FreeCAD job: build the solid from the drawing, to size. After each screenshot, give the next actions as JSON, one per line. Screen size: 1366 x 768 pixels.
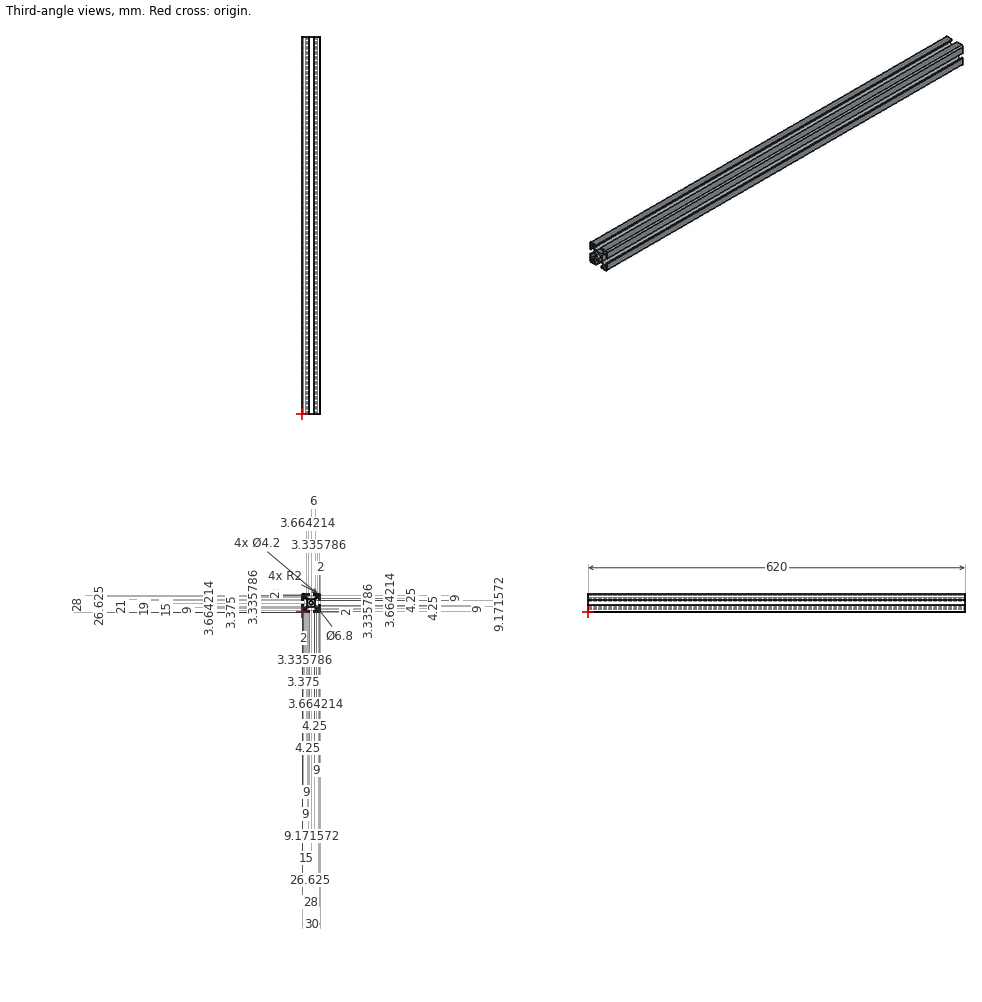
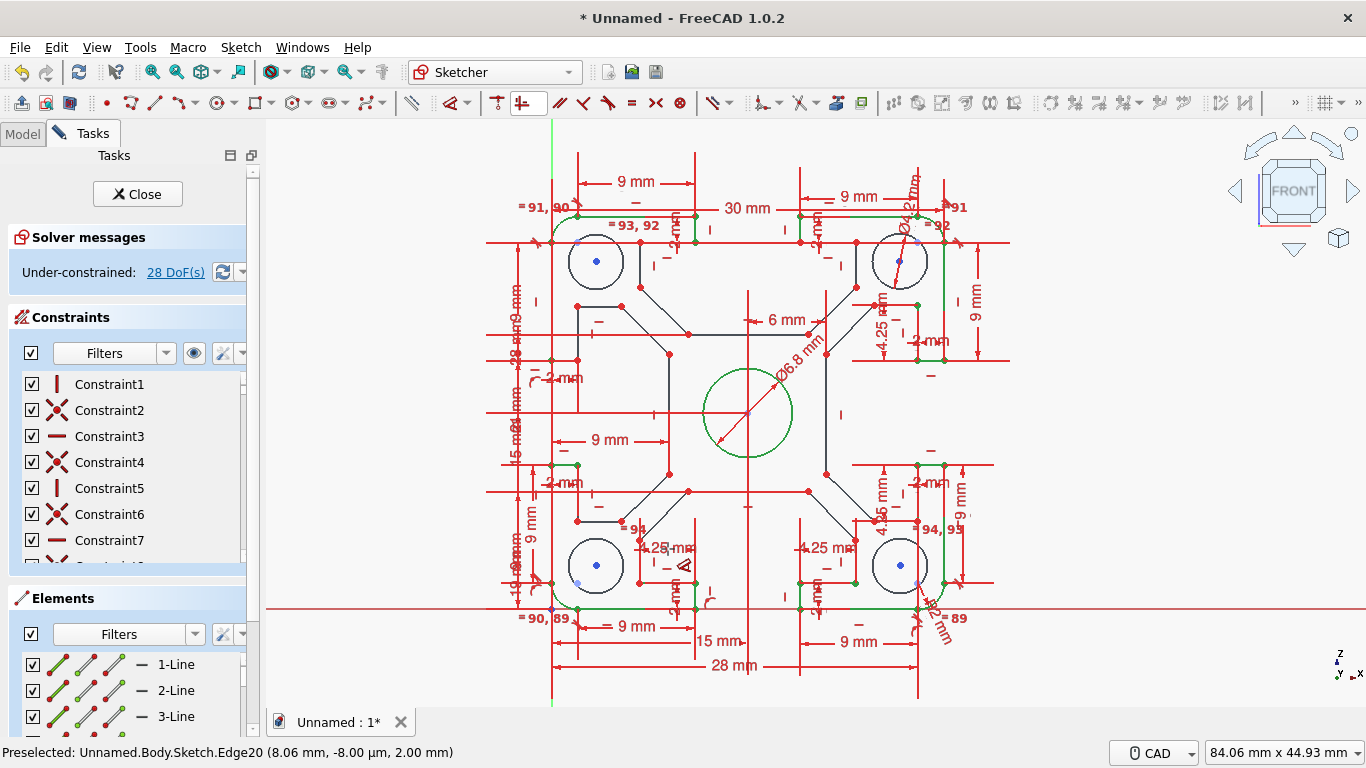
{"action": "left_click", "coordinate": [578, 482]}
{"action": "left_click", "coordinate": [612, 506]}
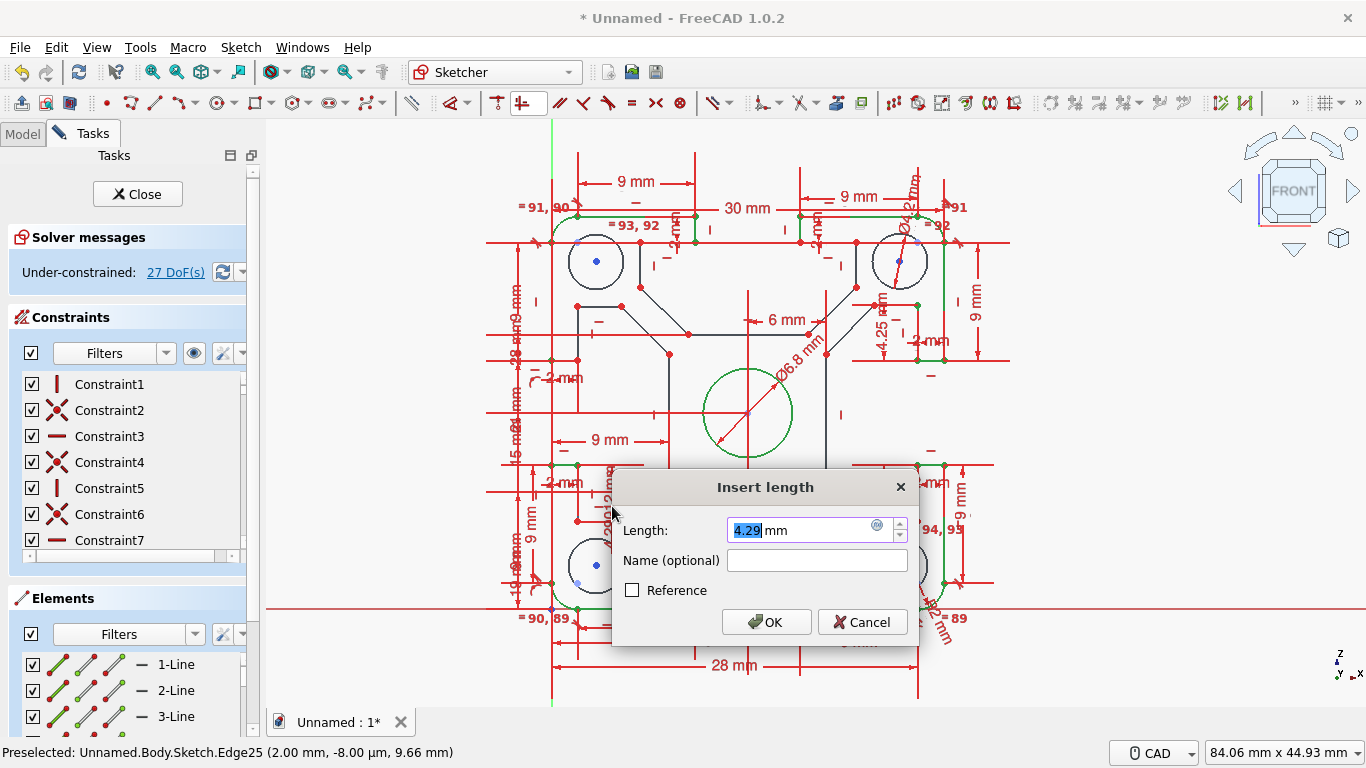
{"action": "type", "text": "4.25"}
{"action": "key", "text": "Return"}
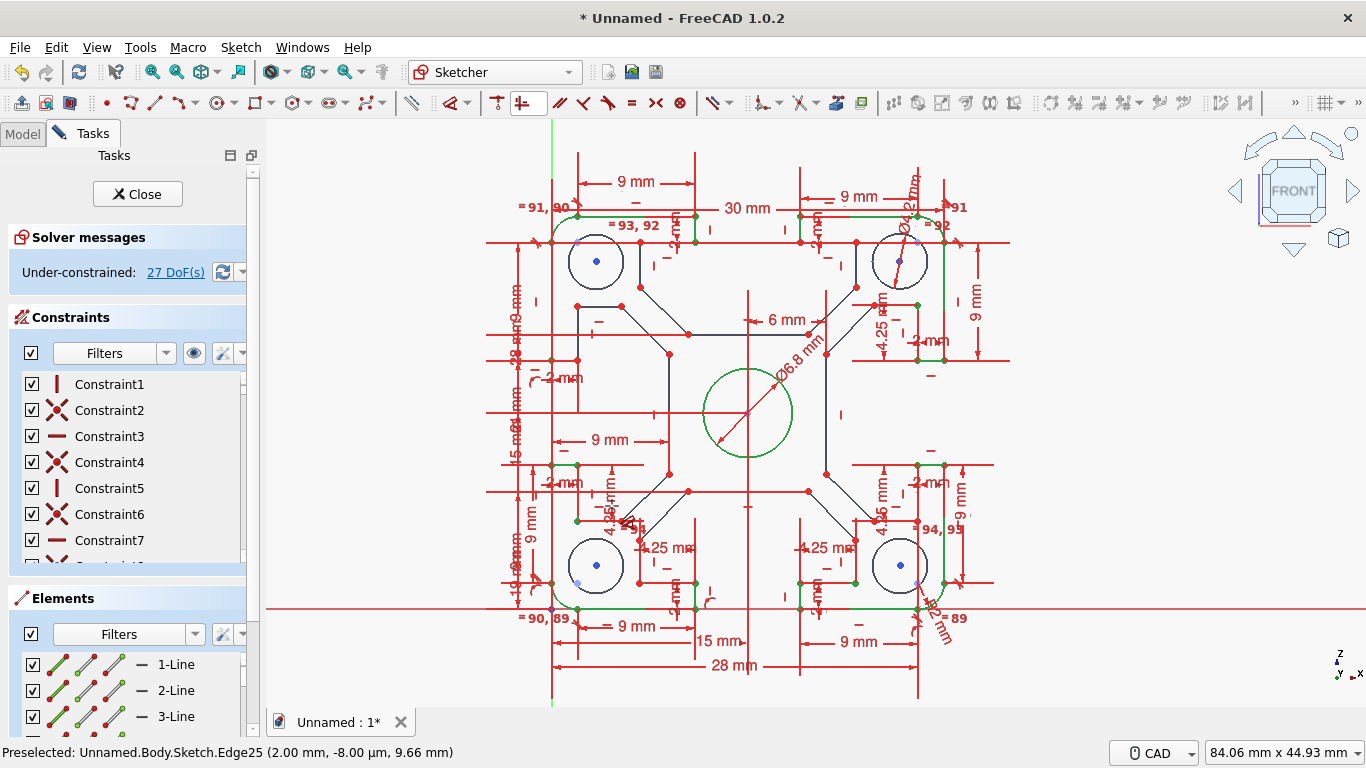
{"action": "left_click", "coordinate": [578, 323]}
{"action": "left_click", "coordinate": [612, 334]}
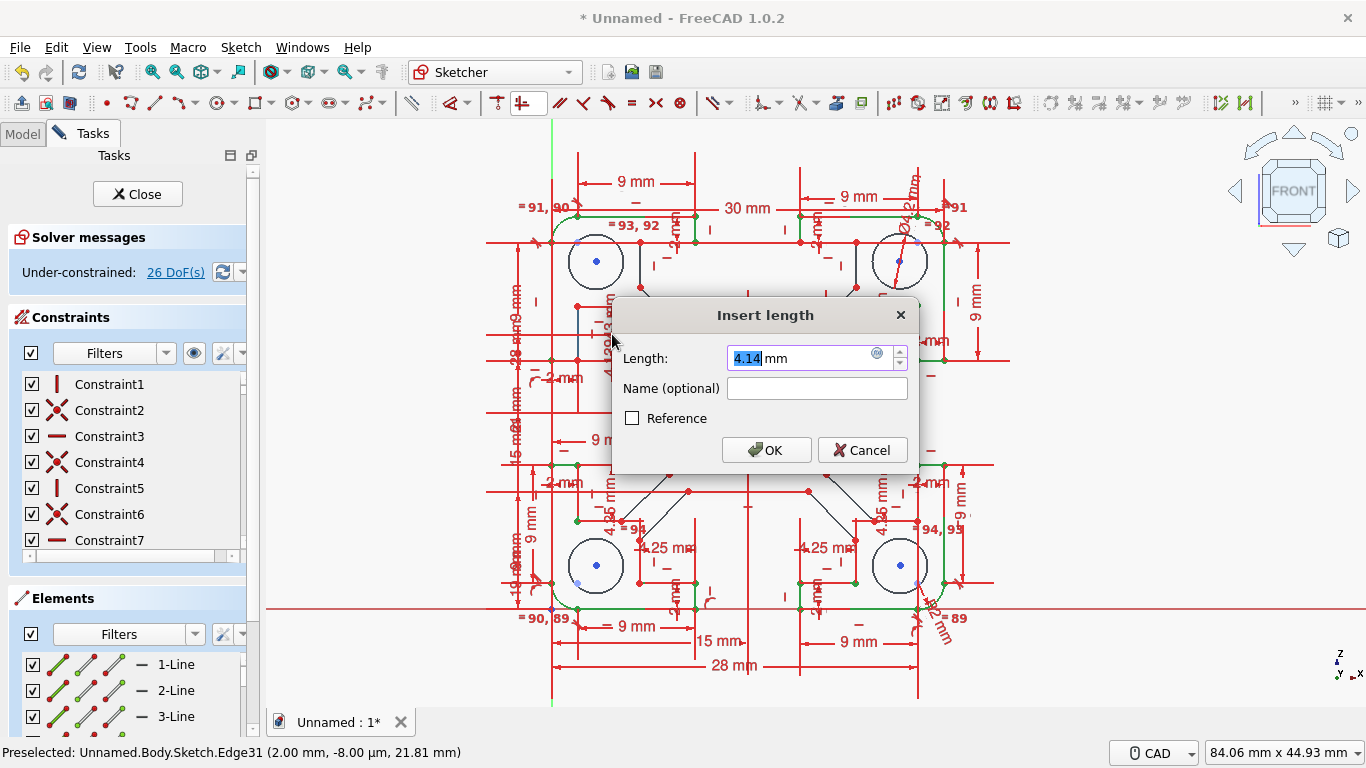
{"action": "type", "text": "4.25"}
{"action": "key", "text": "Return"}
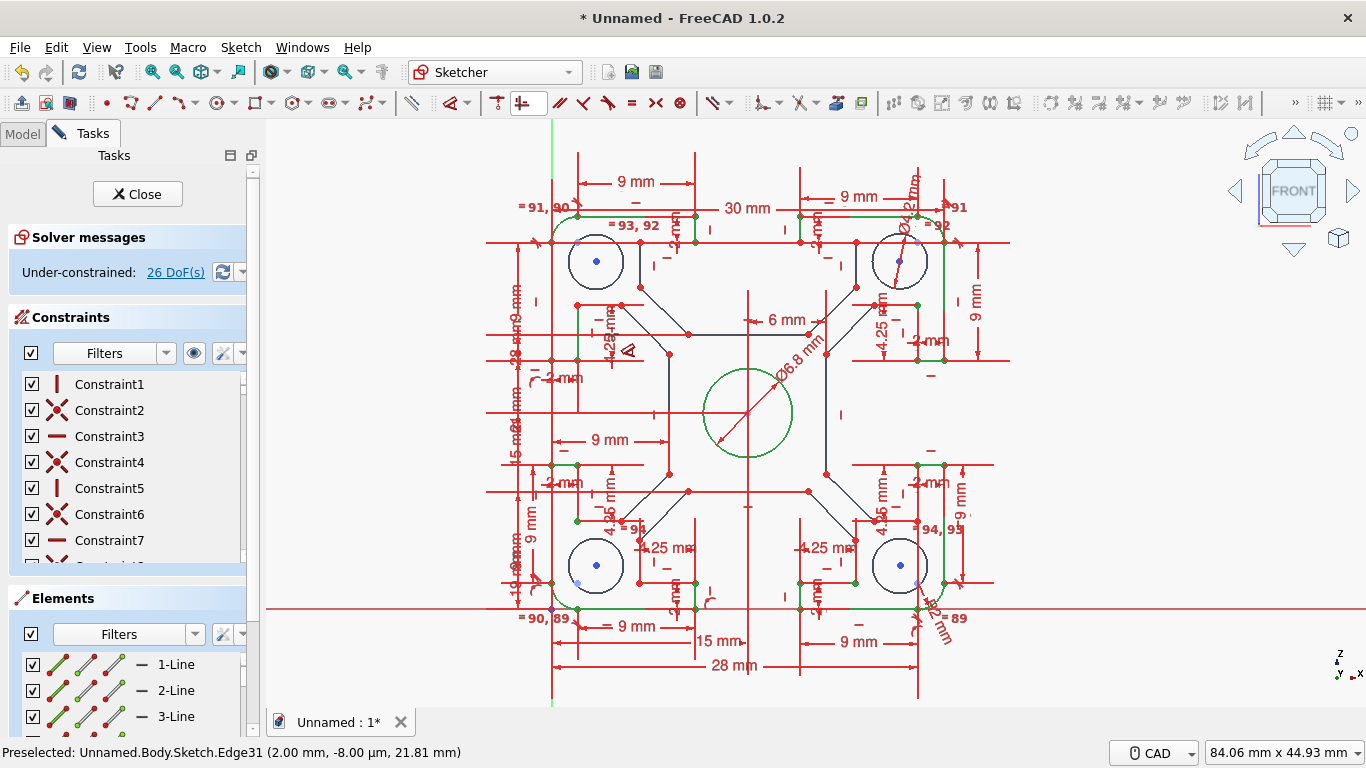
{"action": "left_click", "coordinate": [679, 243]}
{"action": "left_click", "coordinate": [668, 277]}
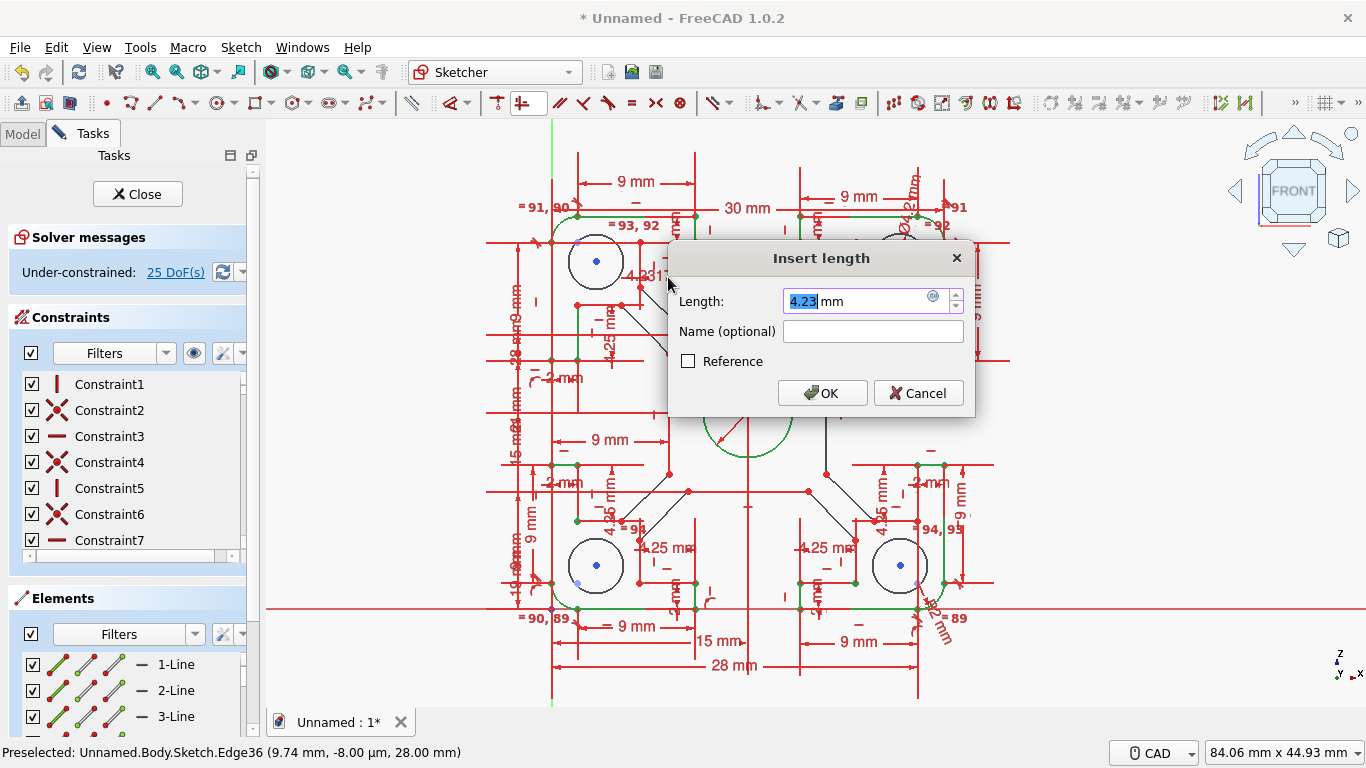
{"action": "type", "text": "4.25"}
{"action": "key", "text": "Return"}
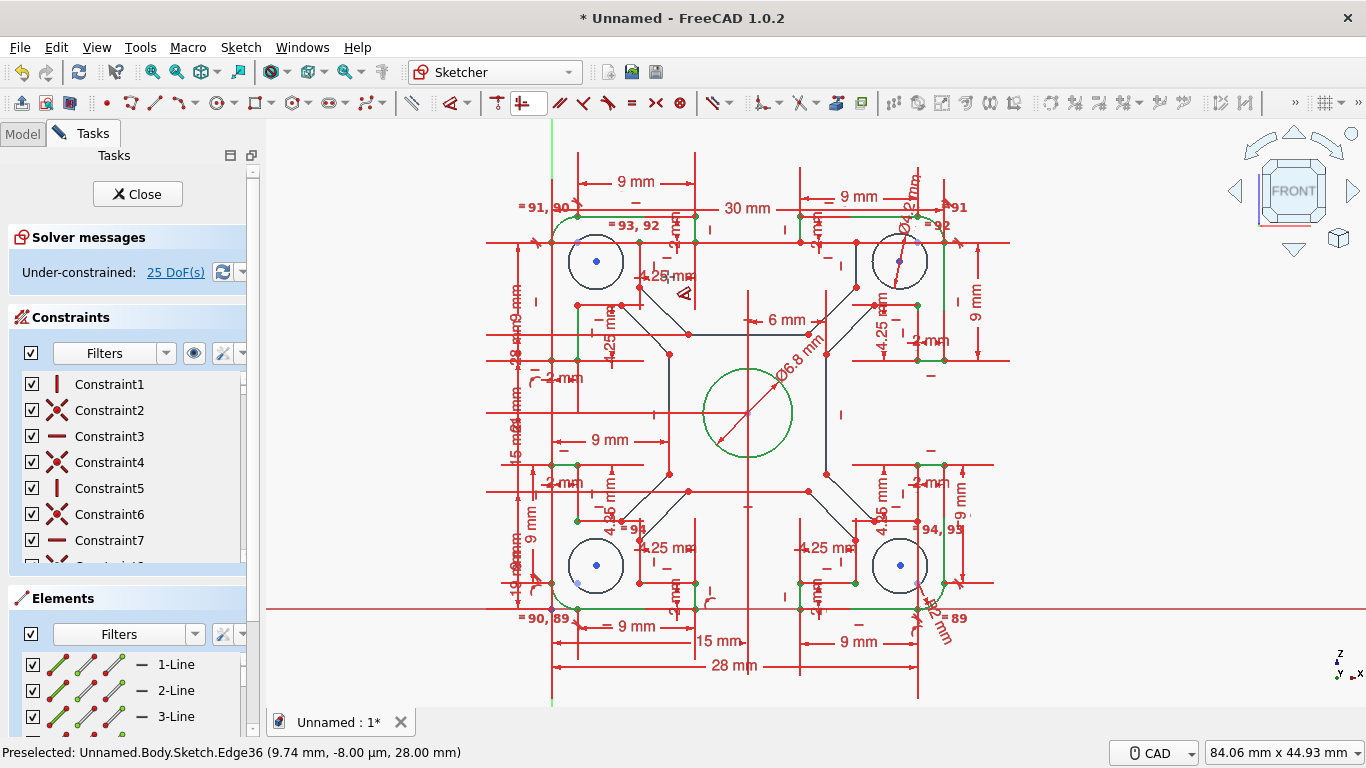
{"action": "left_click", "coordinate": [839, 243]}
{"action": "left_click", "coordinate": [828, 277]}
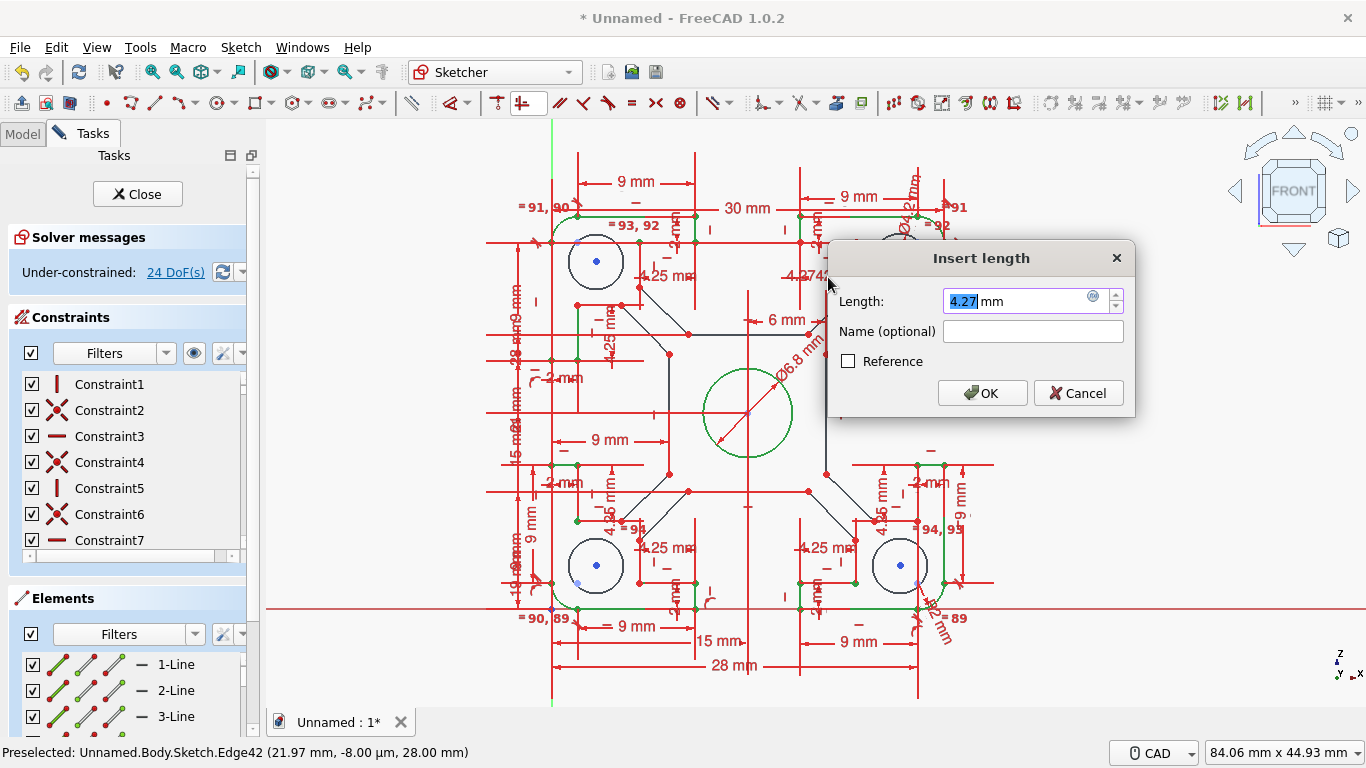
{"action": "type", "text": "4.25"}
{"action": "key", "text": "Return"}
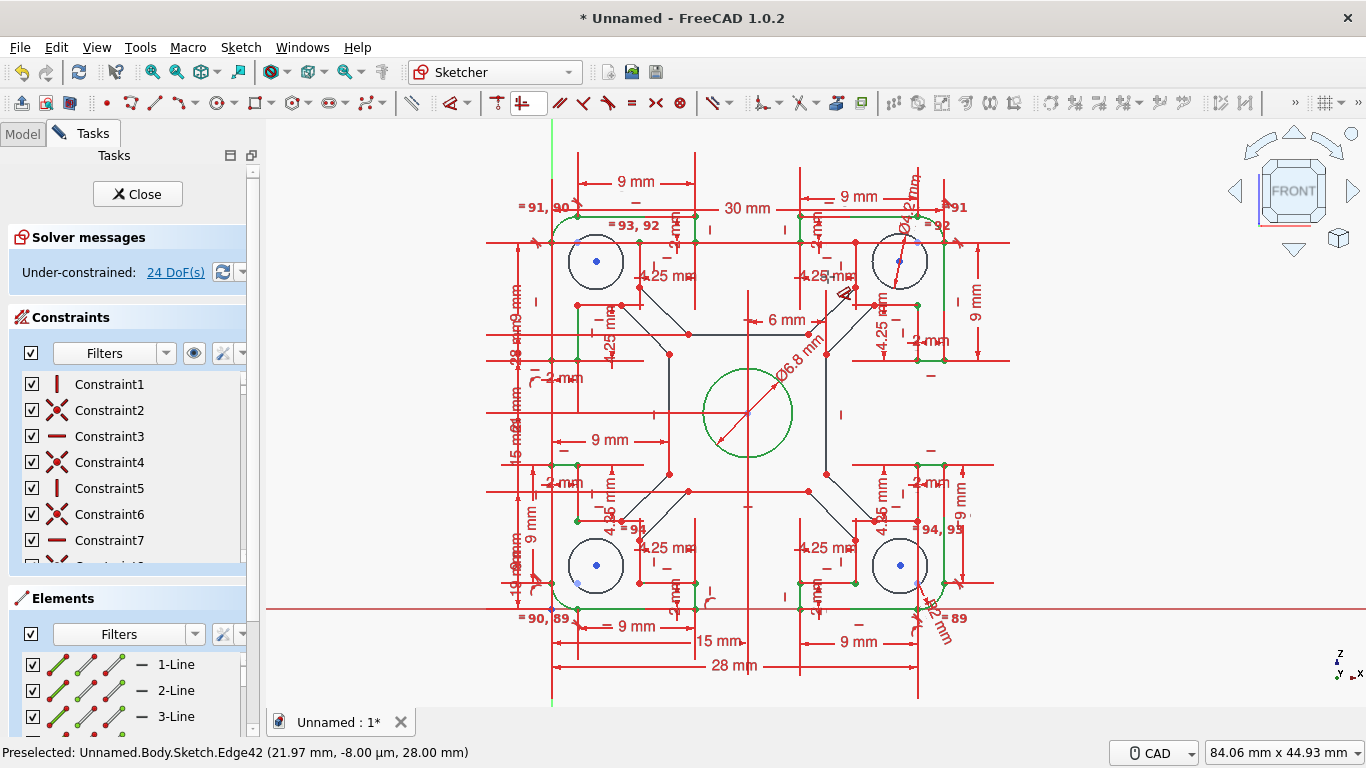
{"action": "left_click", "coordinate": [596, 262]}
{"action": "left_click", "coordinate": [574, 667]}